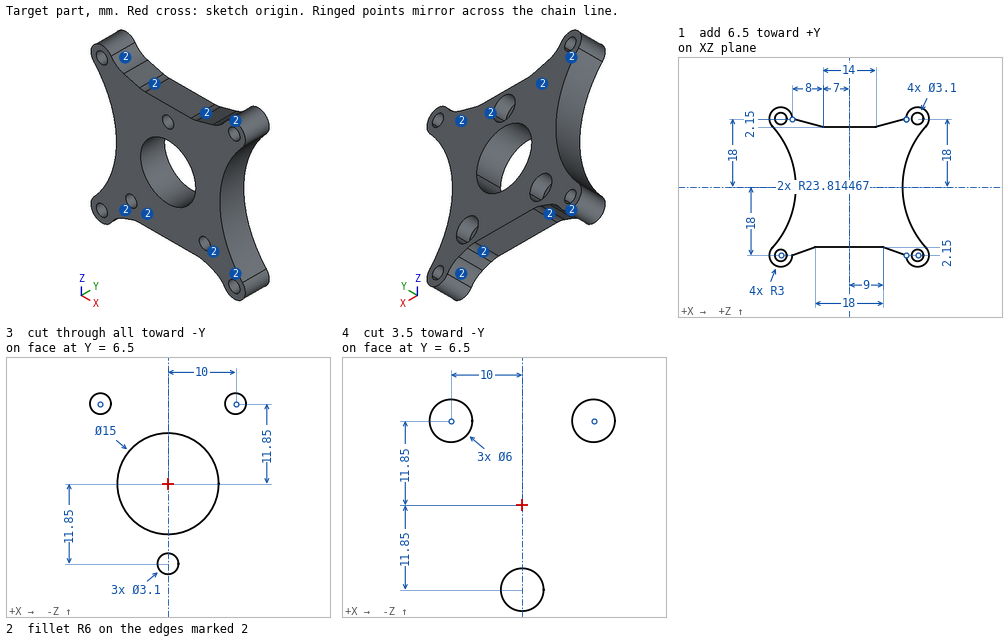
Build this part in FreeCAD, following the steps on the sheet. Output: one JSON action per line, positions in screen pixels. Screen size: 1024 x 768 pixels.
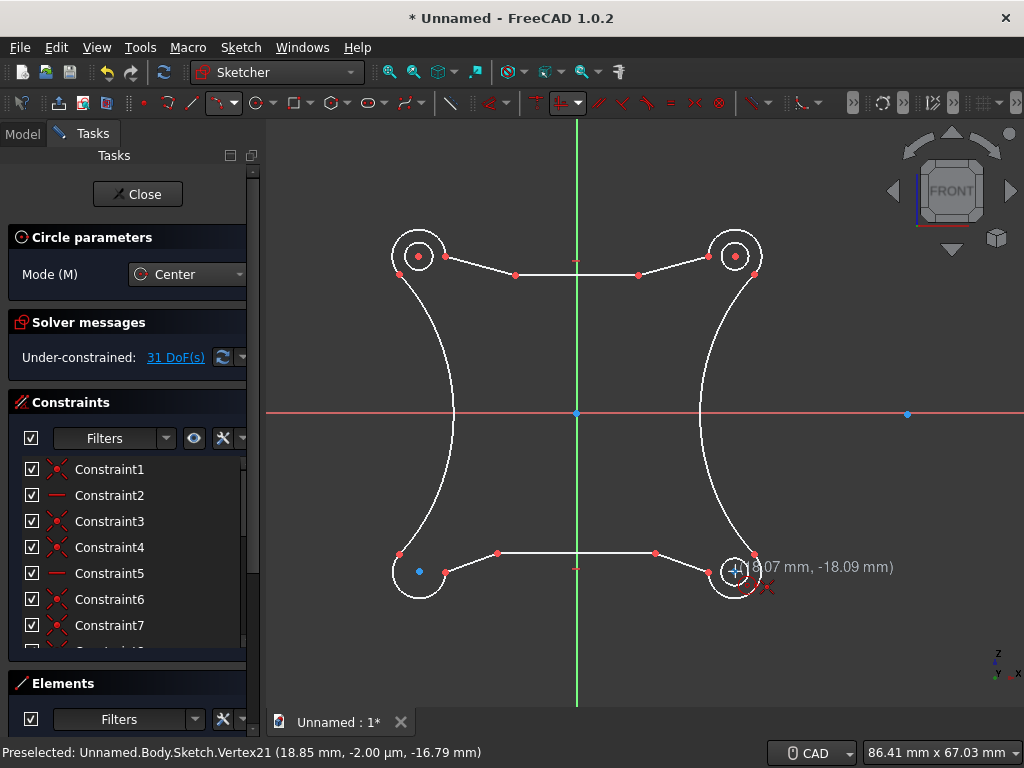
{"action": "scroll", "coordinate": [419, 571], "scroll_direction": "up", "scroll_amount": 3}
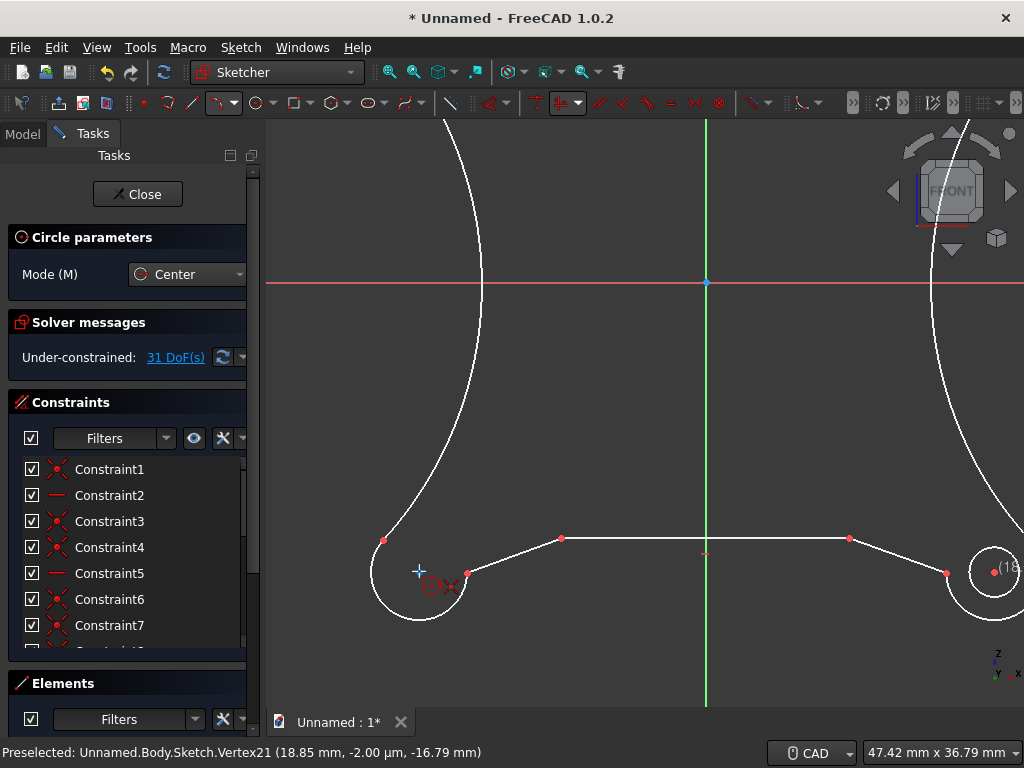
{"action": "left_click", "coordinate": [419, 571]}
{"action": "left_click", "coordinate": [436, 553]}
{"action": "key", "text": "Escape"}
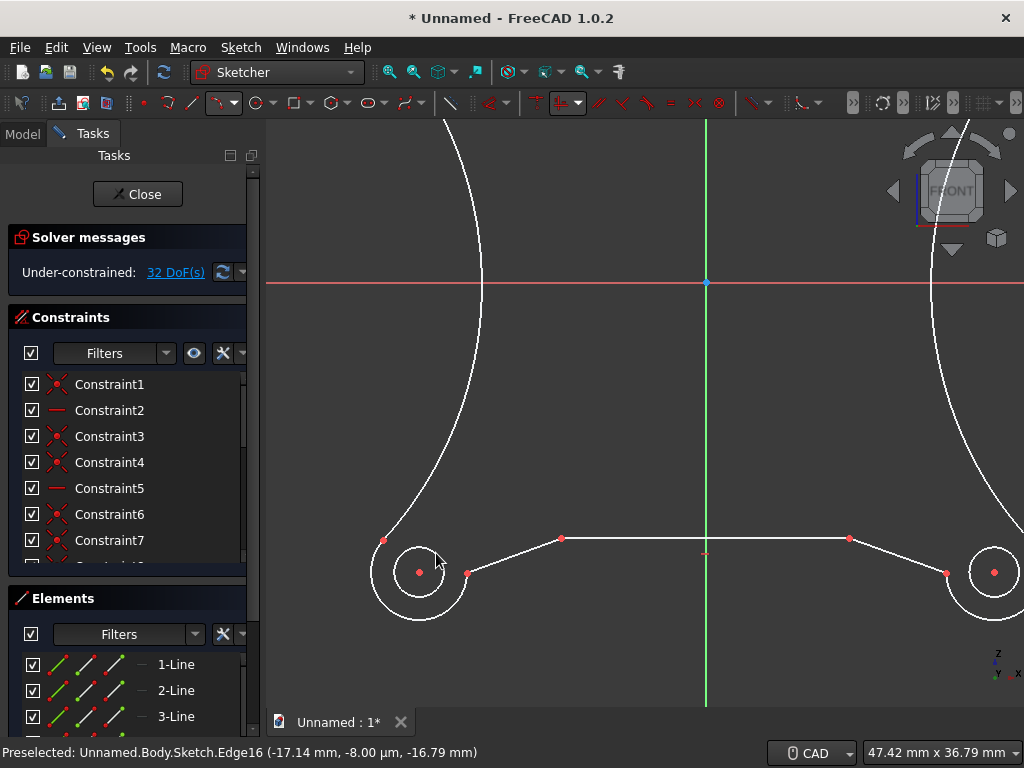
{"action": "scroll", "coordinate": [419, 571], "scroll_direction": "down", "scroll_amount": 3}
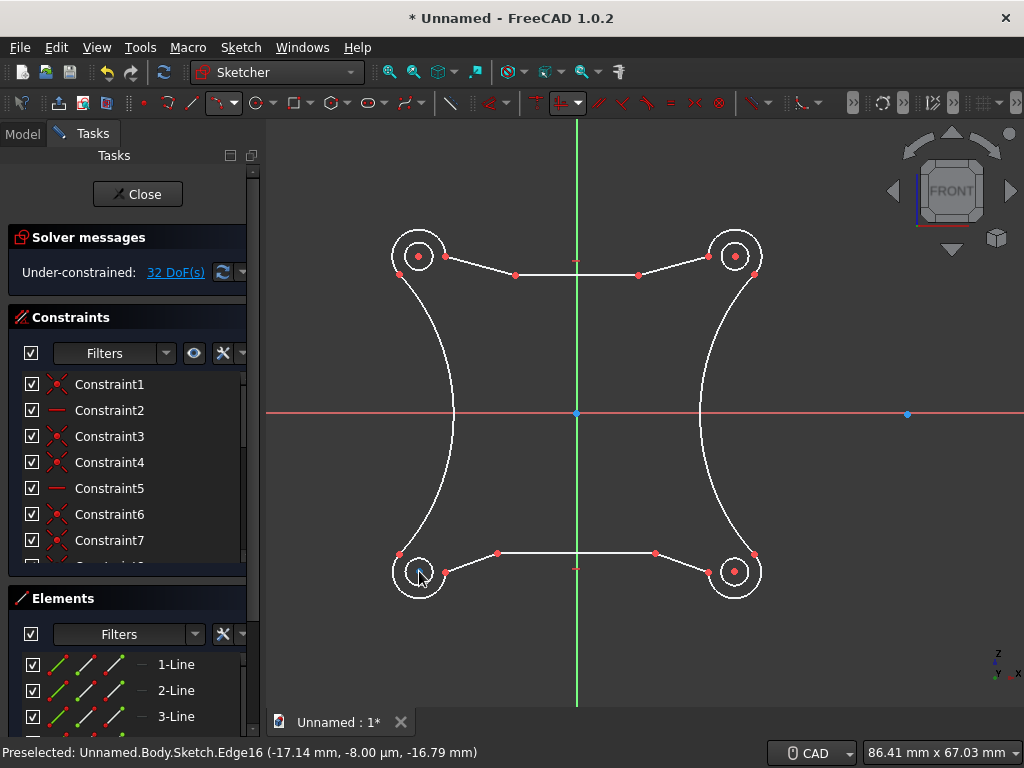
{"action": "left_click", "coordinate": [759, 246]}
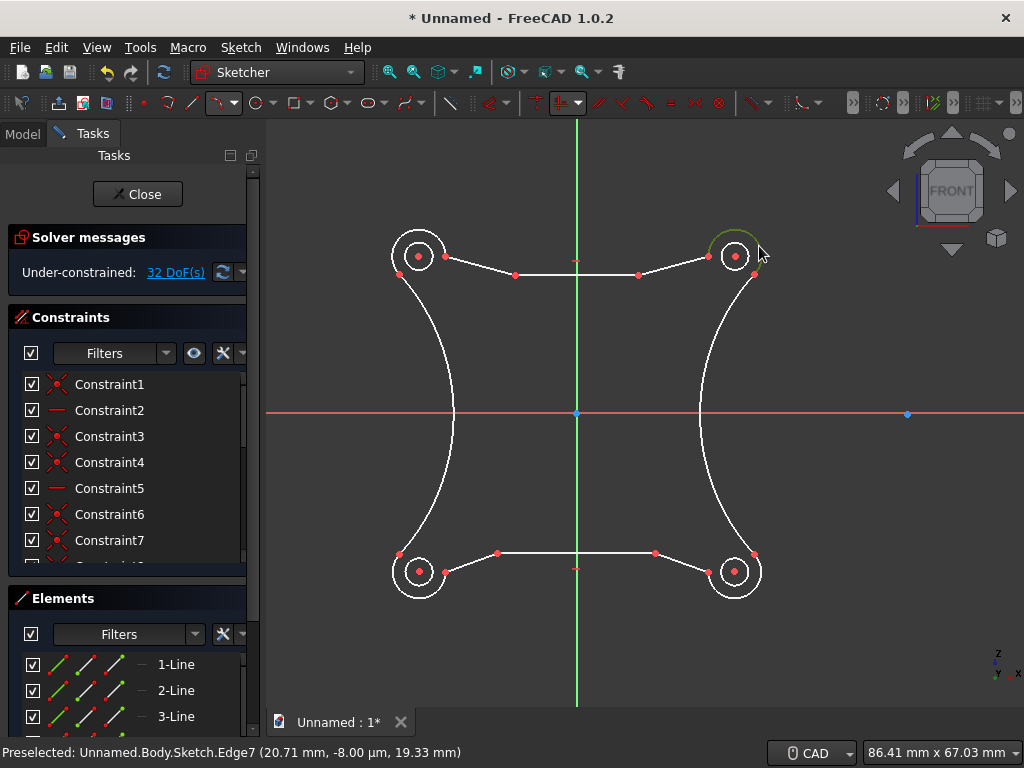
{"action": "left_click", "coordinate": [709, 354]}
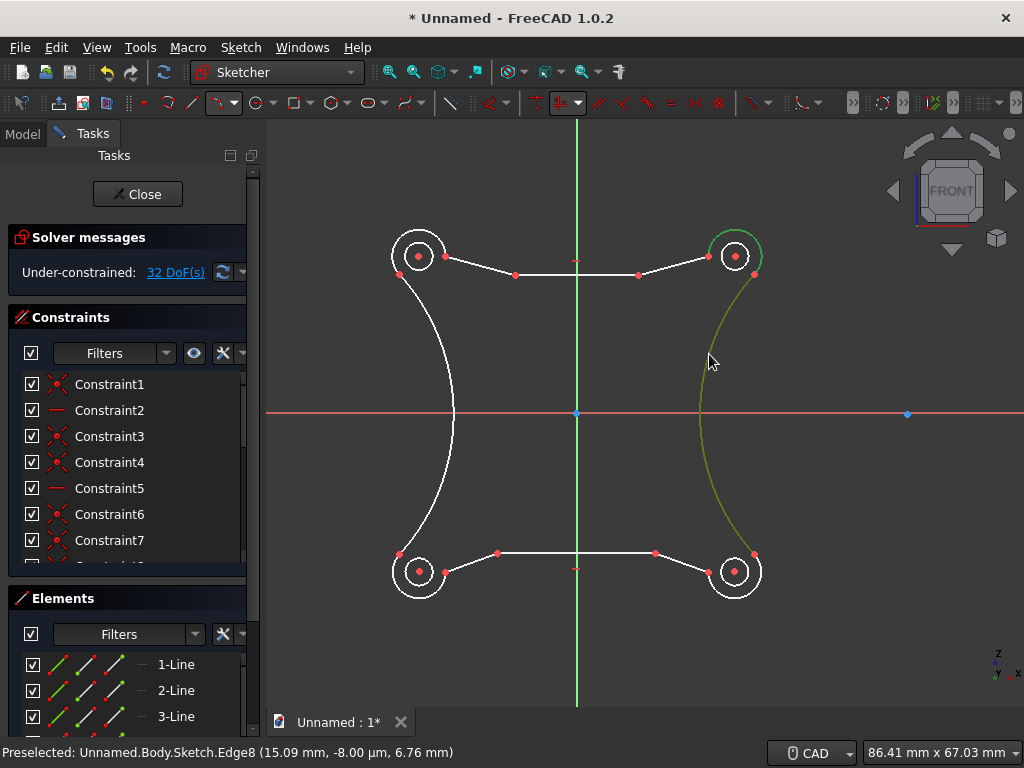
{"action": "left_click", "coordinate": [648, 104]}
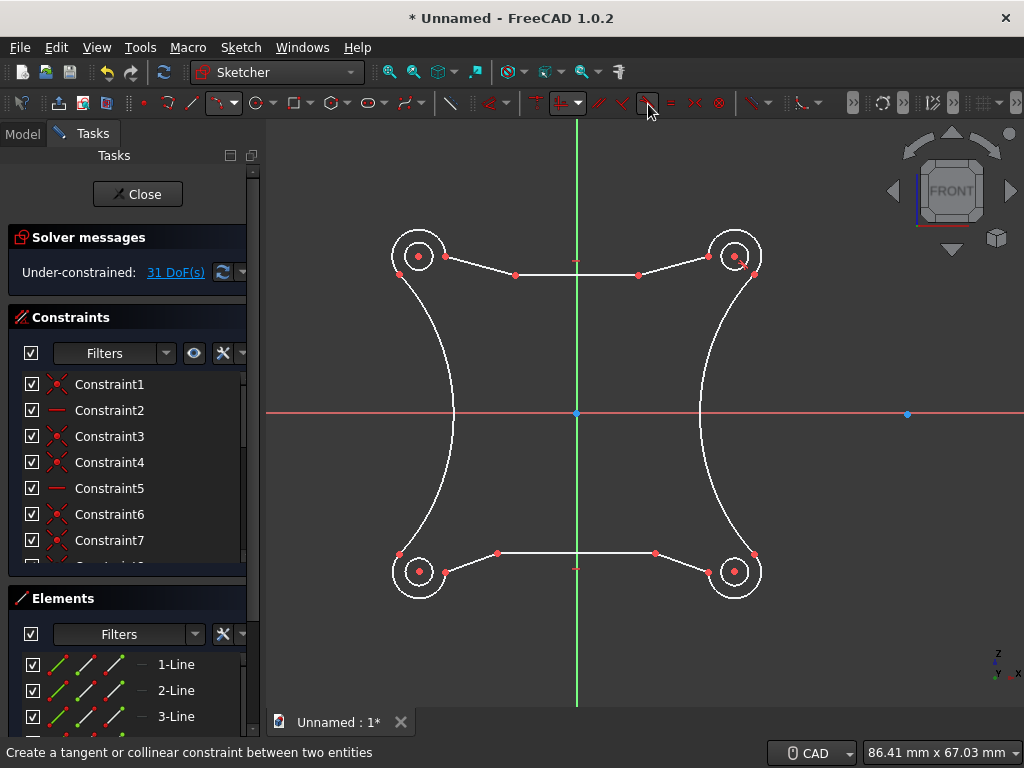
{"action": "left_click", "coordinate": [709, 354]}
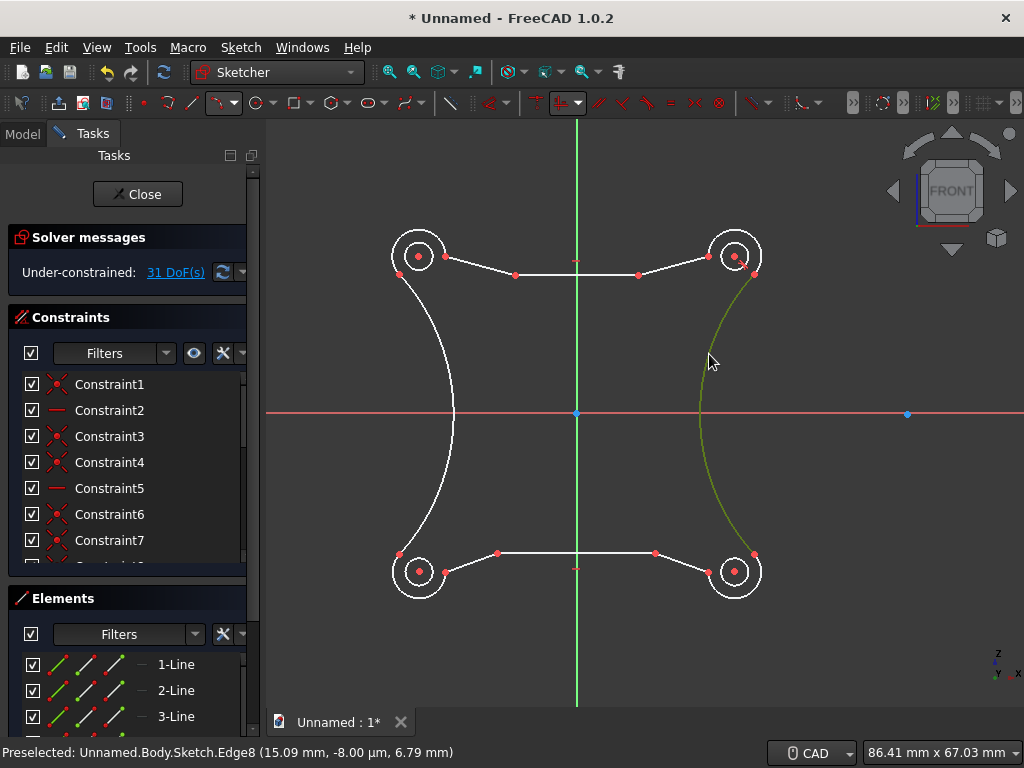
{"action": "left_click", "coordinate": [725, 596]}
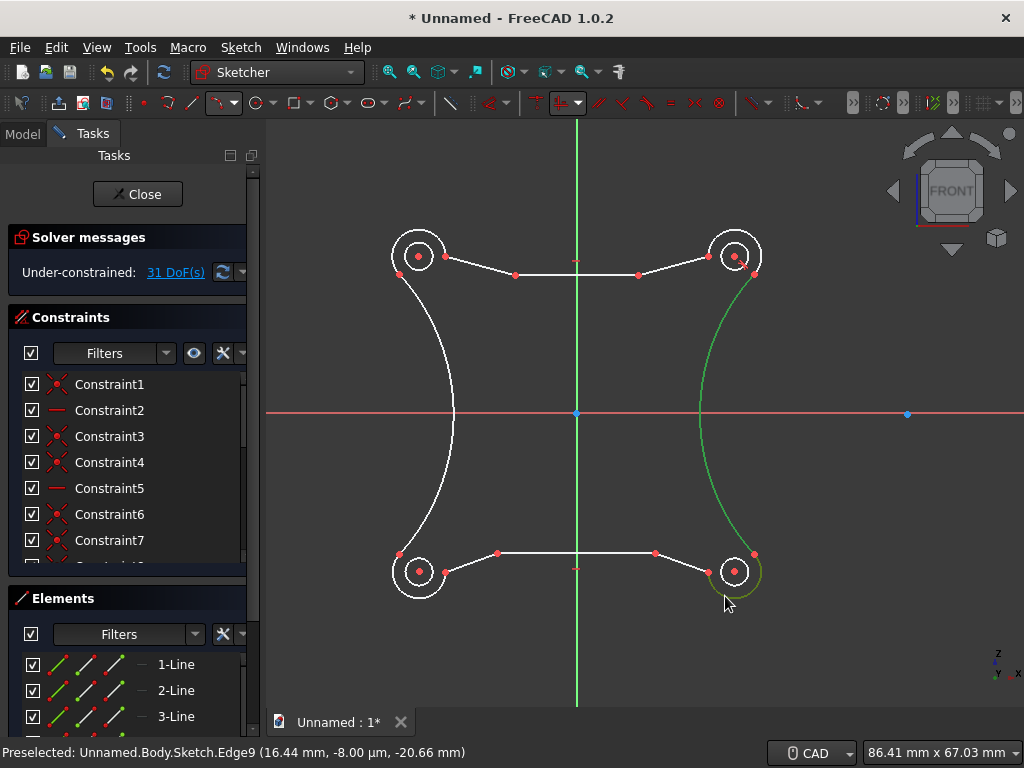
{"action": "left_click", "coordinate": [648, 104]}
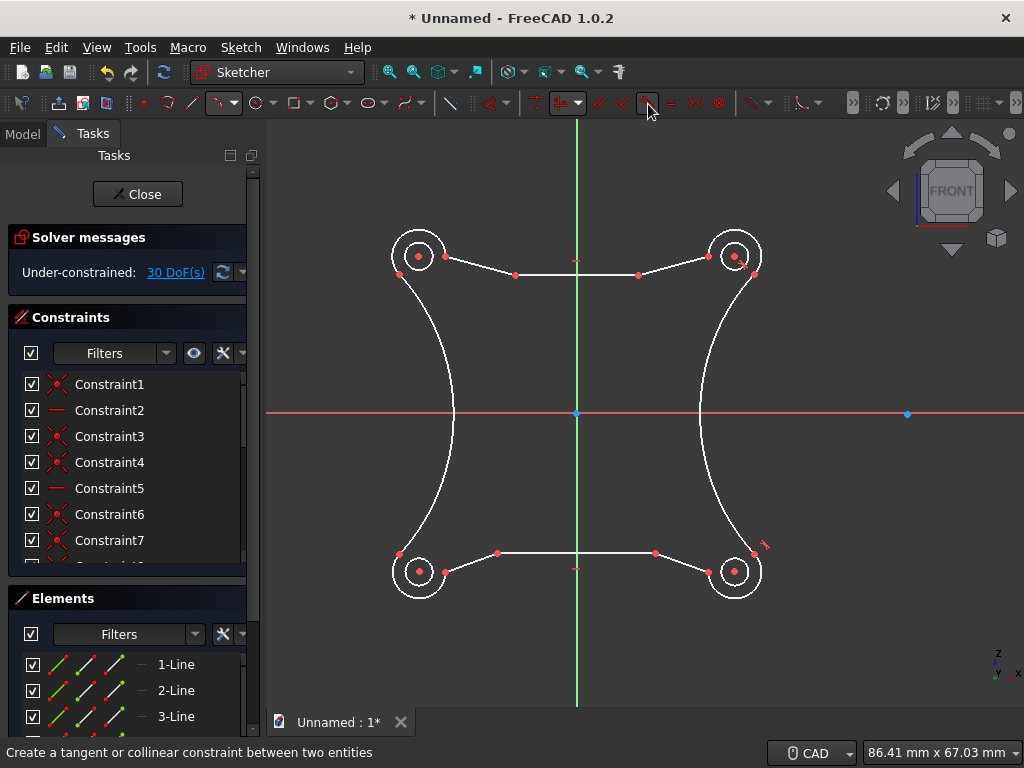
{"action": "left_click", "coordinate": [395, 583]}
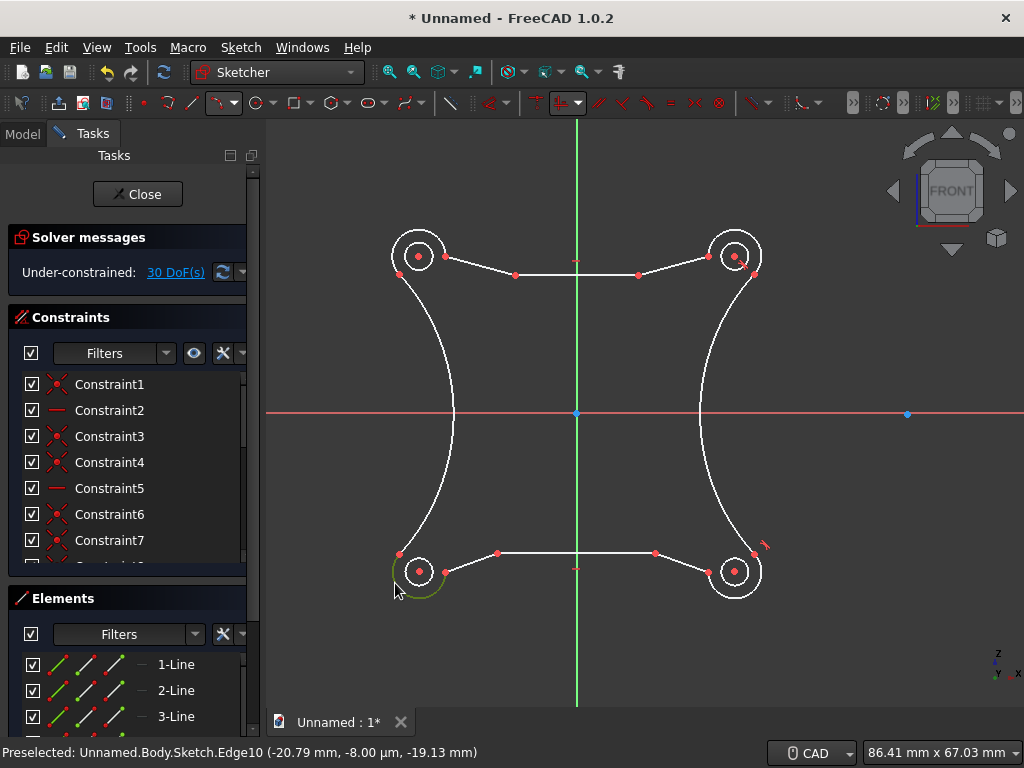
{"action": "left_click", "coordinate": [445, 475]}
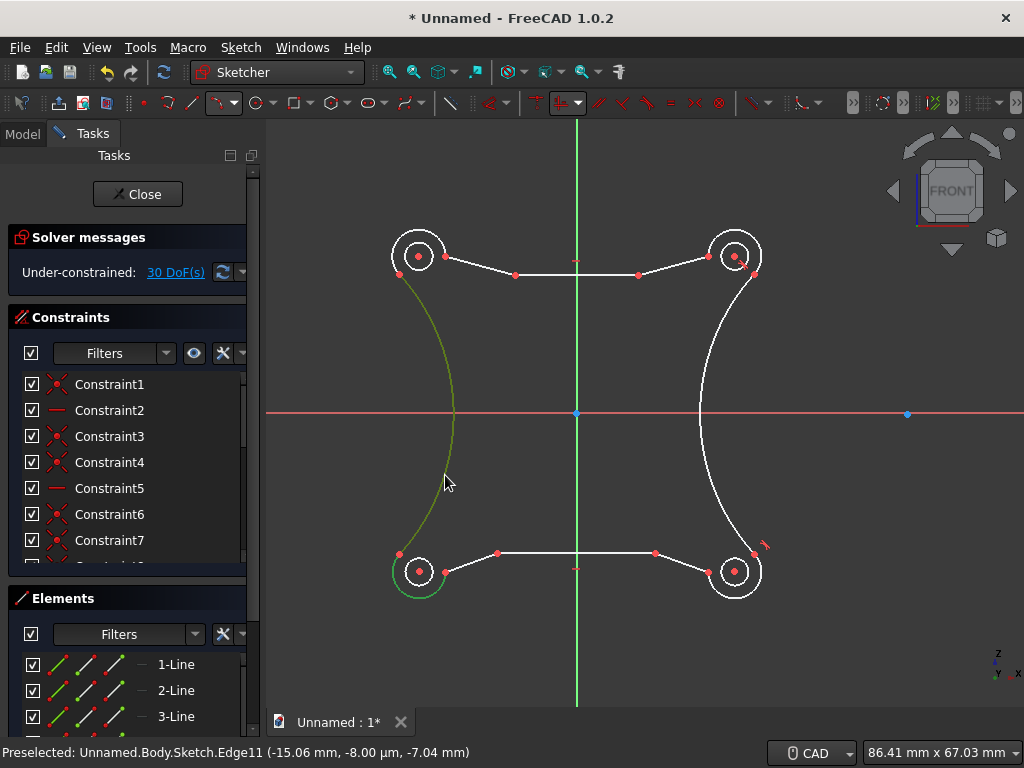
{"action": "left_click", "coordinate": [648, 104]}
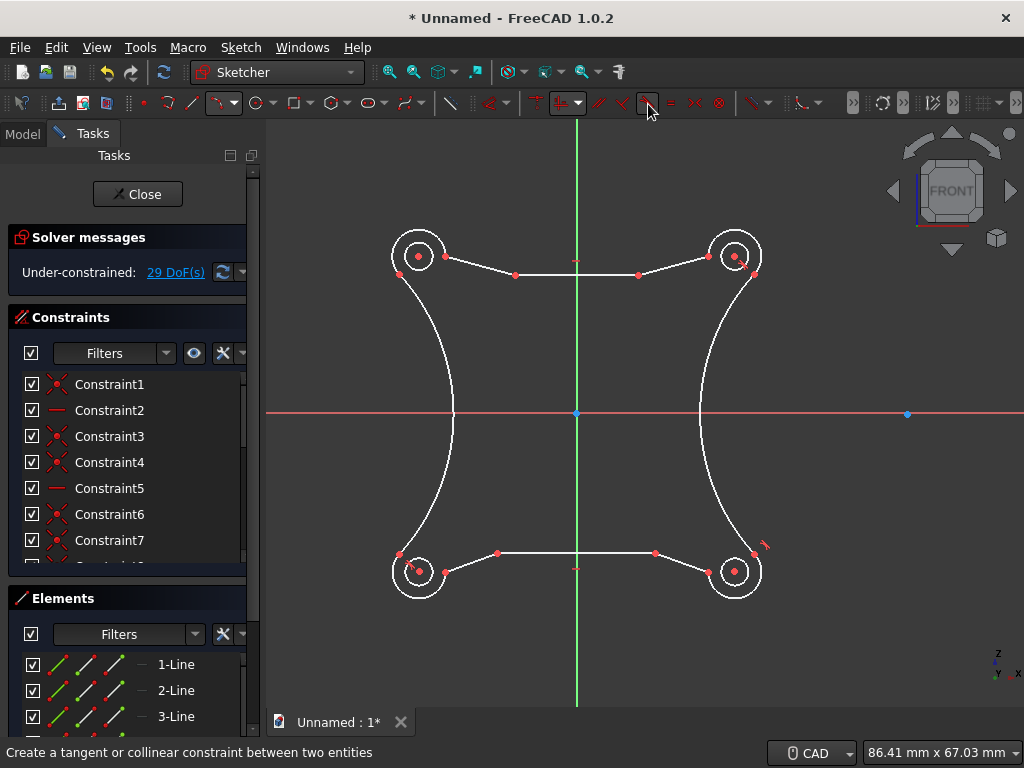
{"action": "left_click", "coordinate": [445, 475]}